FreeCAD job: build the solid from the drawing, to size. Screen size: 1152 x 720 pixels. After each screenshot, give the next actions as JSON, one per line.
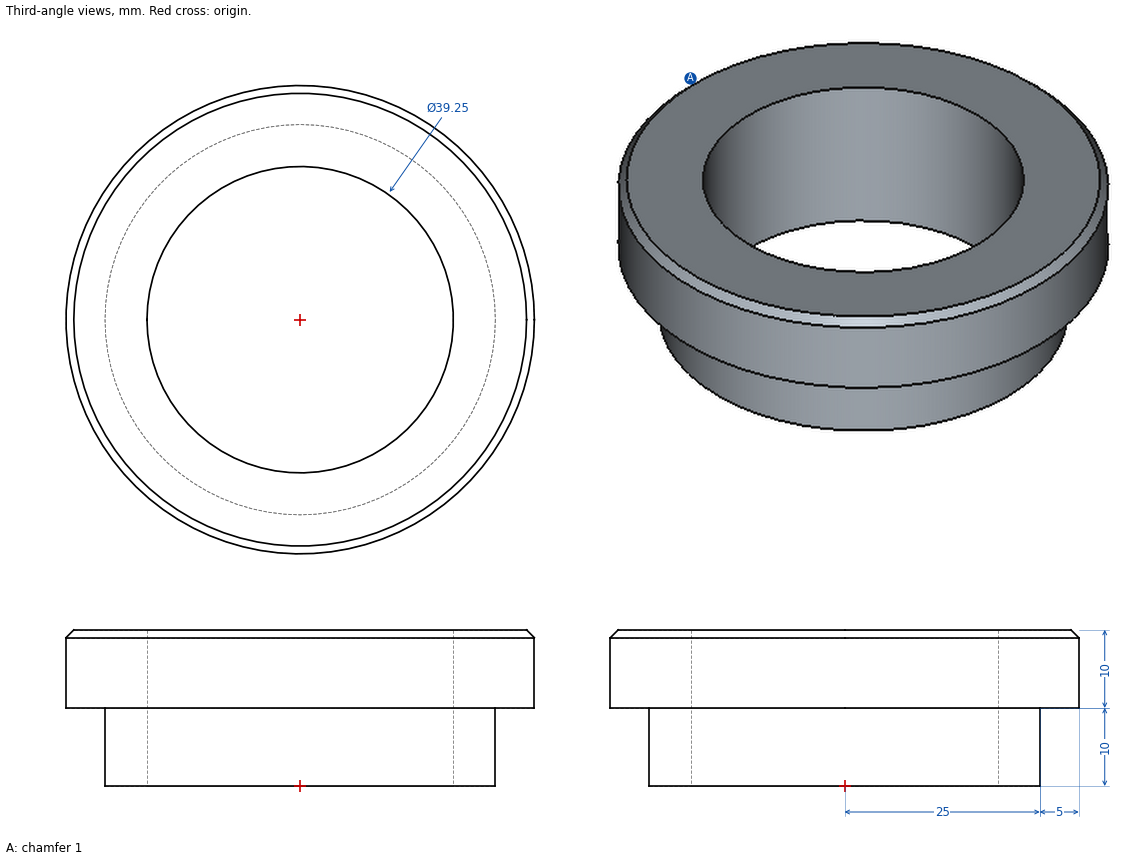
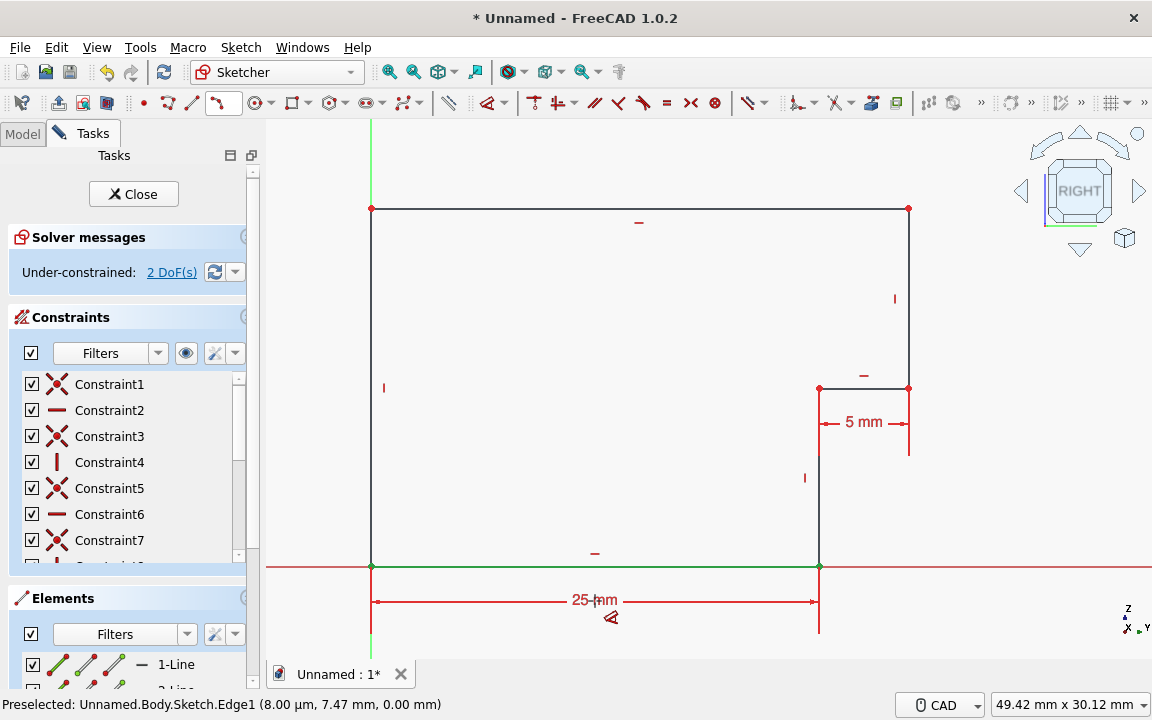
{"action": "left_click", "coordinate": [819, 513]}
{"action": "left_click", "coordinate": [853, 478]}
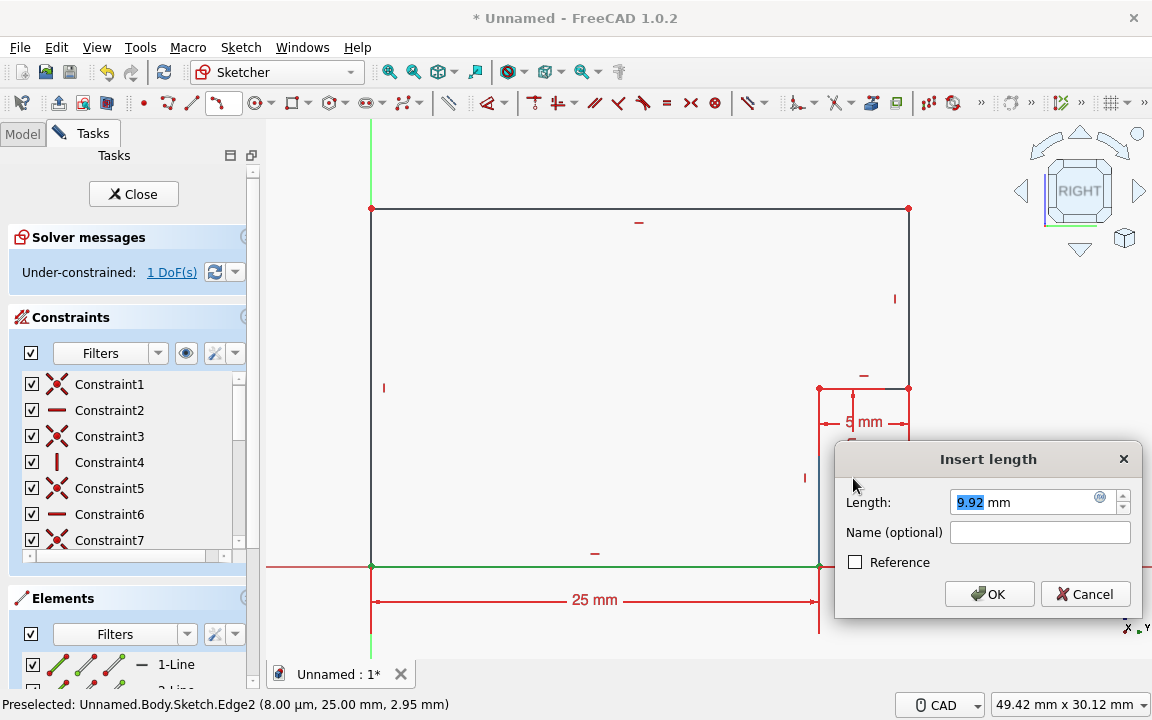
{"action": "type", "text": "10"}
{"action": "key", "text": "Return"}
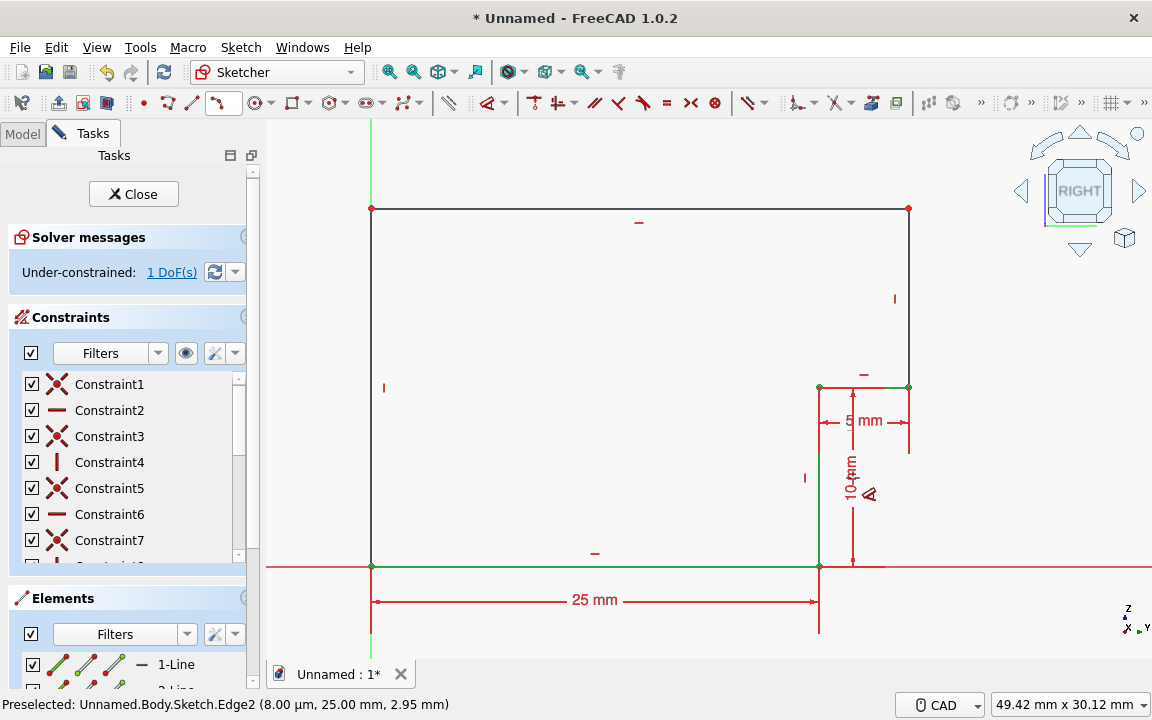
{"action": "left_click", "coordinate": [909, 334]}
{"action": "left_click", "coordinate": [943, 298]}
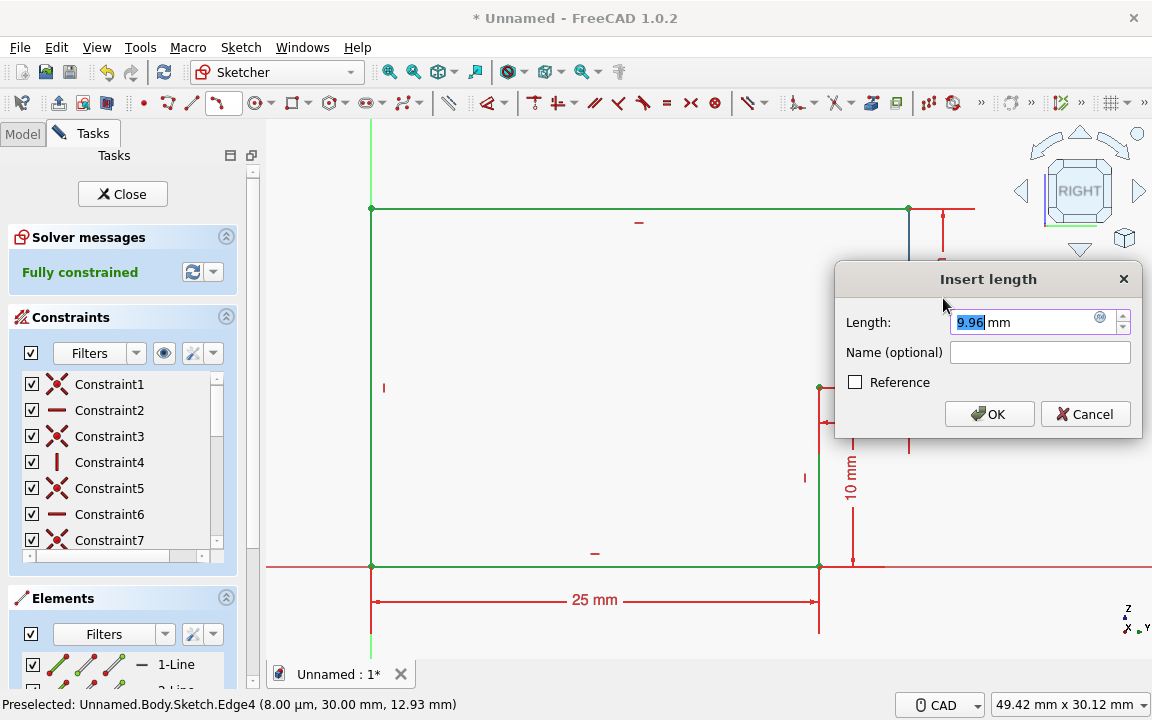
{"action": "type", "text": "10"}
{"action": "key", "text": "Return"}
{"action": "key", "text": "Escape"}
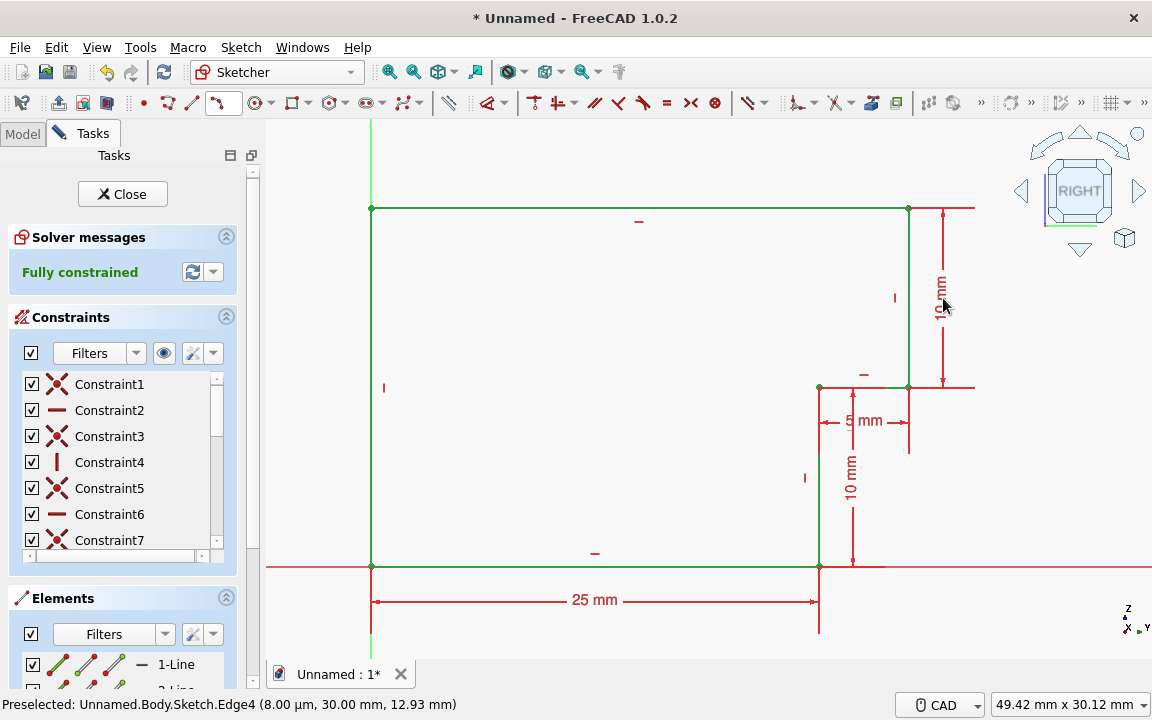
{"action": "left_click", "coordinate": [123, 194]}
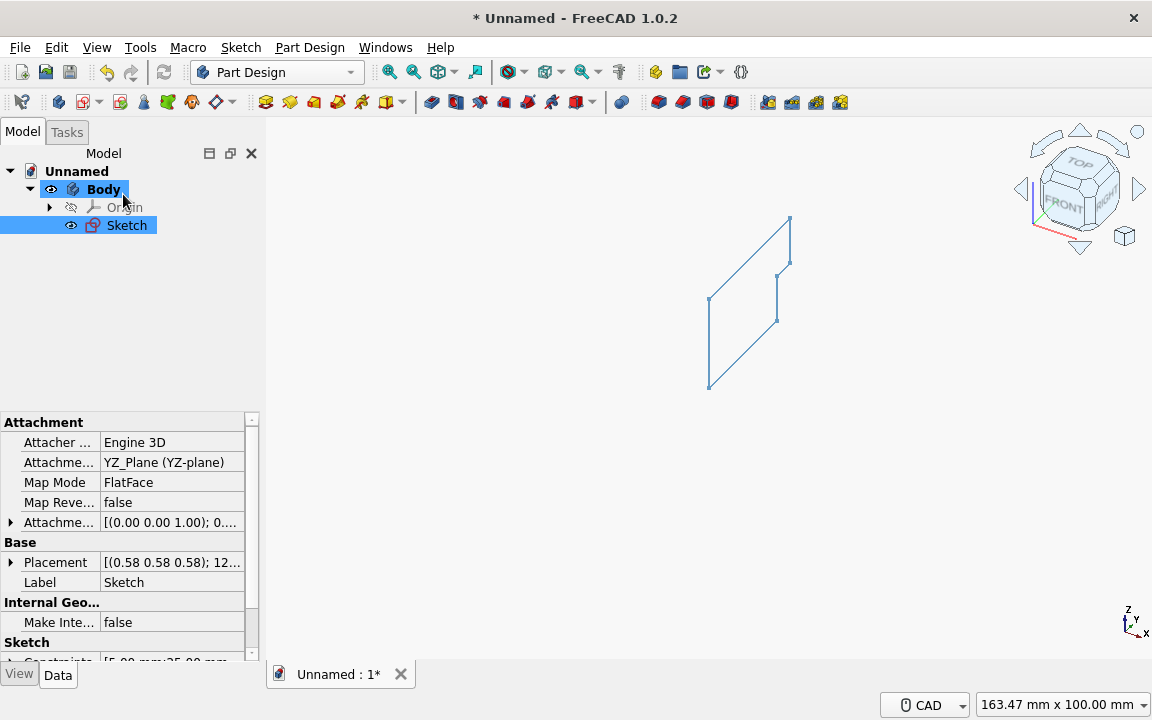
{"action": "left_click", "coordinate": [290, 102]}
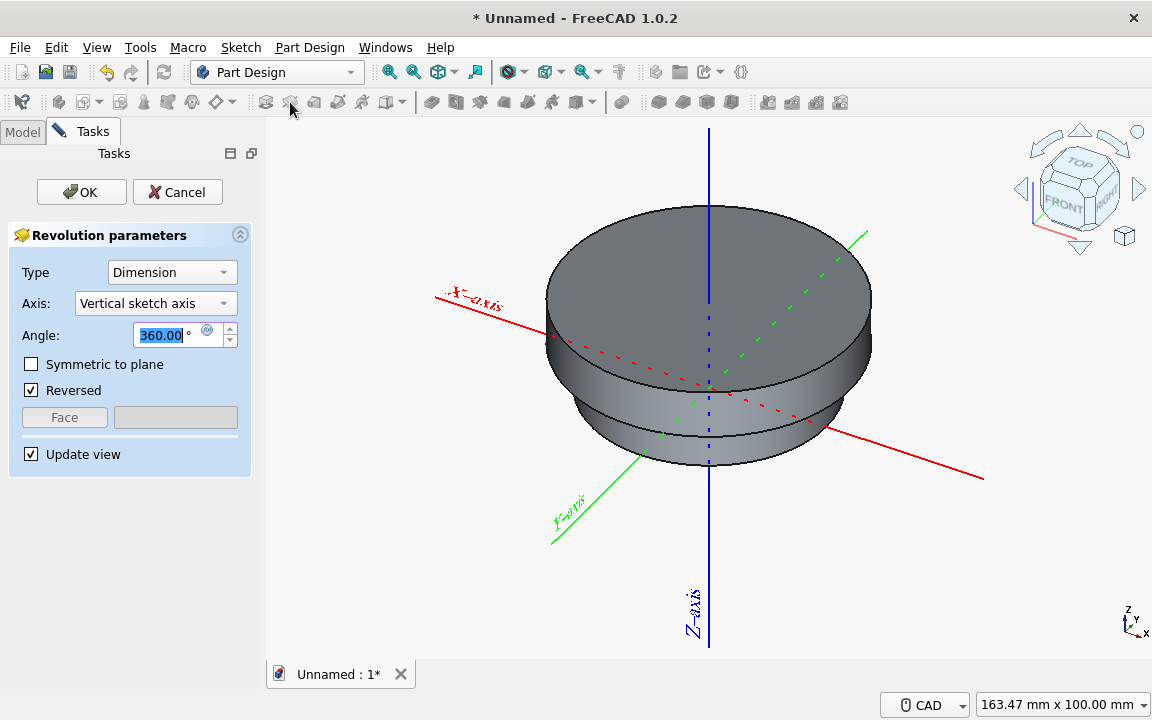
{"action": "left_click", "coordinate": [82, 192]}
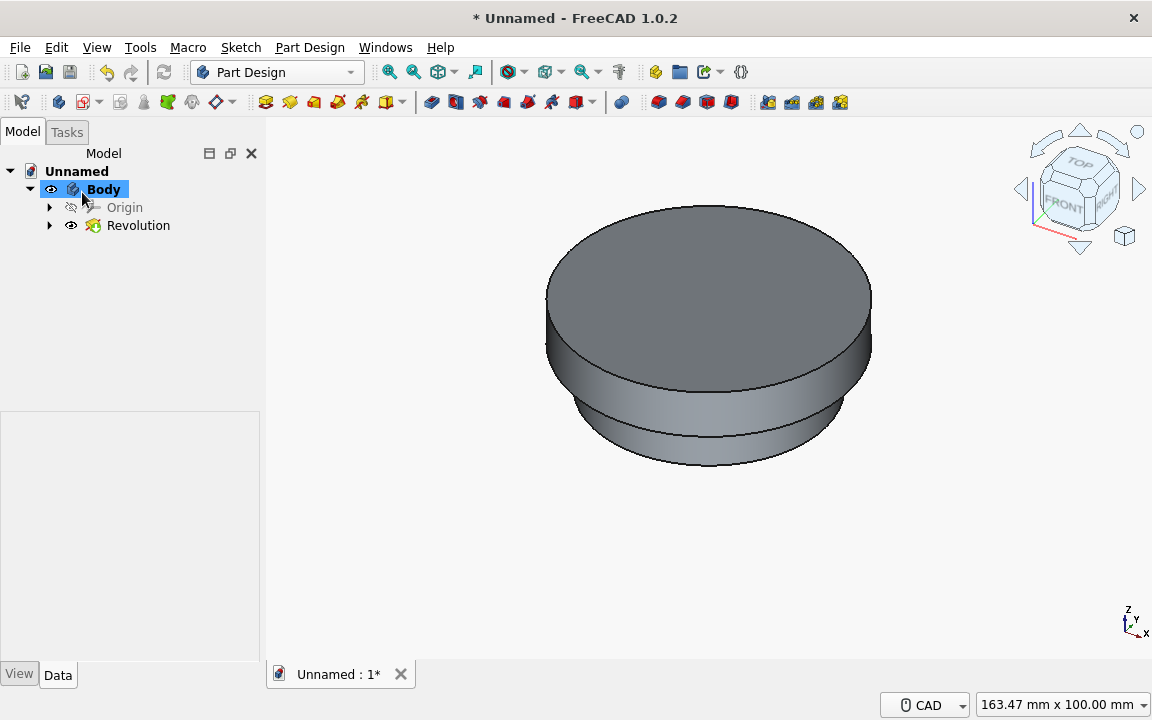
{"action": "left_click", "coordinate": [709, 298]}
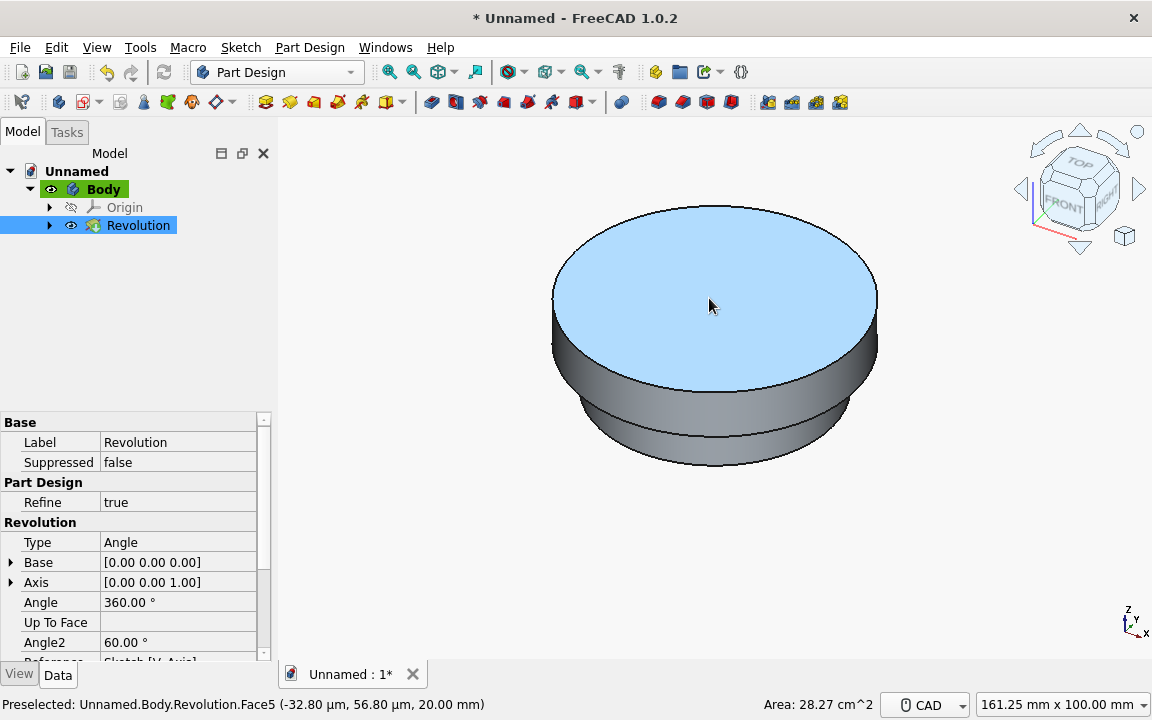
{"action": "left_click", "coordinate": [84, 102]}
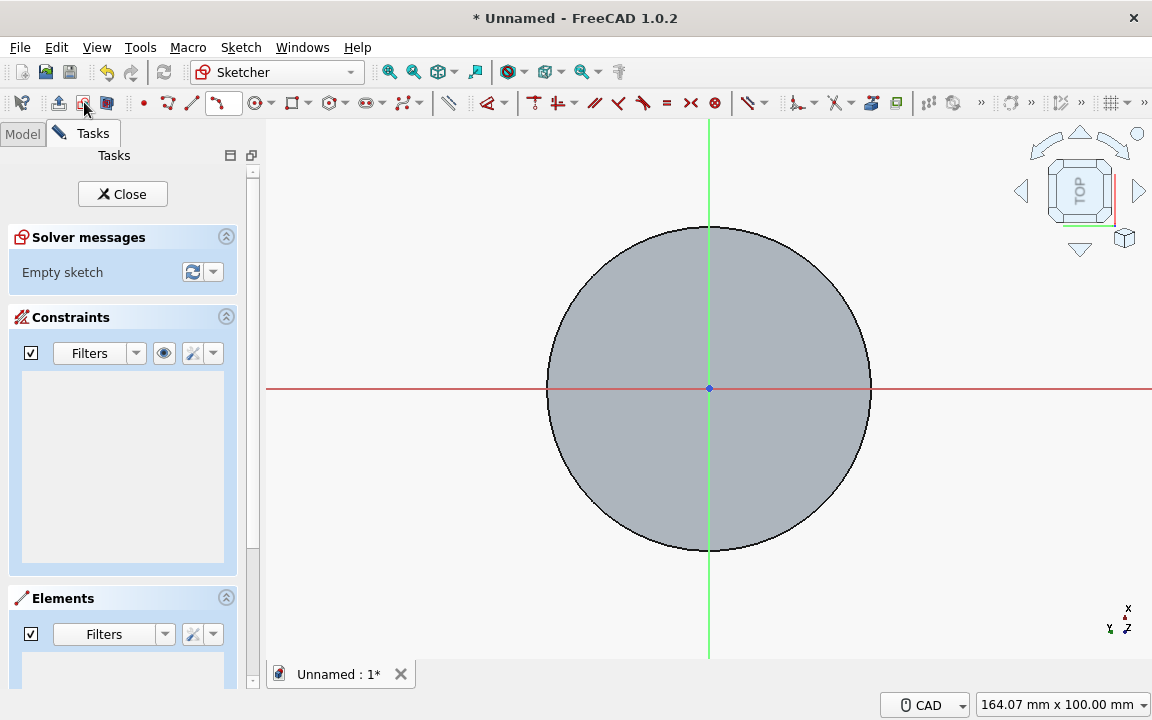
{"action": "scroll", "coordinate": [848, 389], "scroll_direction": "up", "scroll_amount": 2}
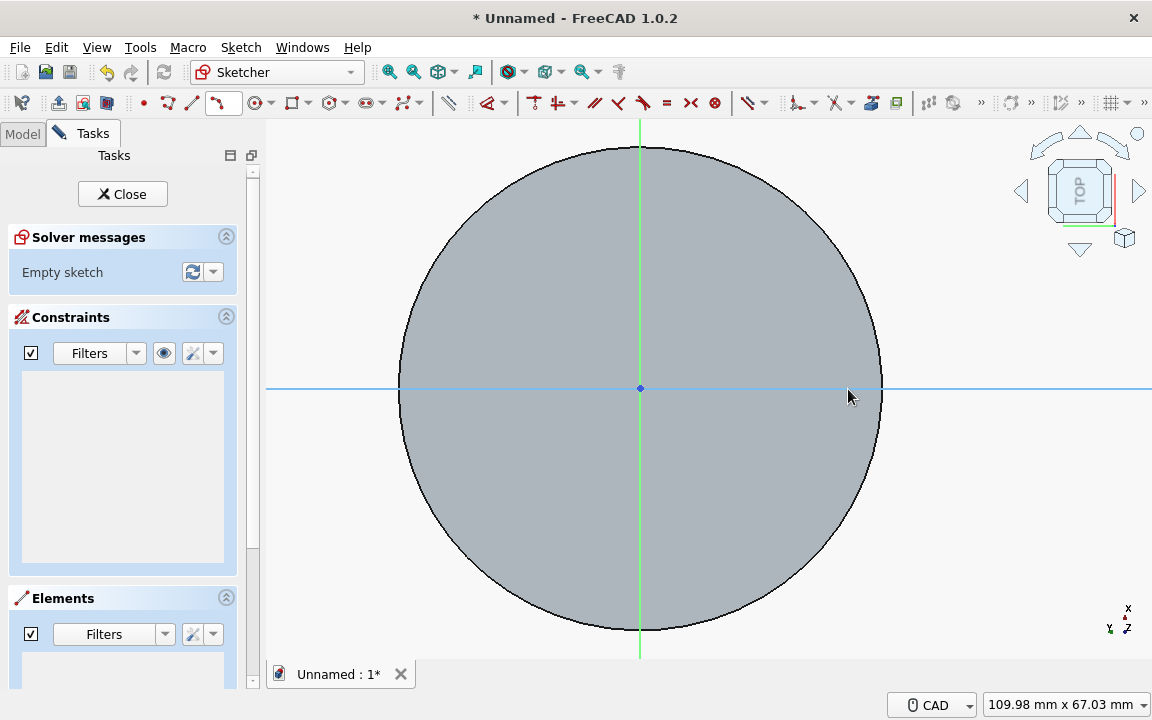
{"action": "left_click", "coordinate": [256, 104]}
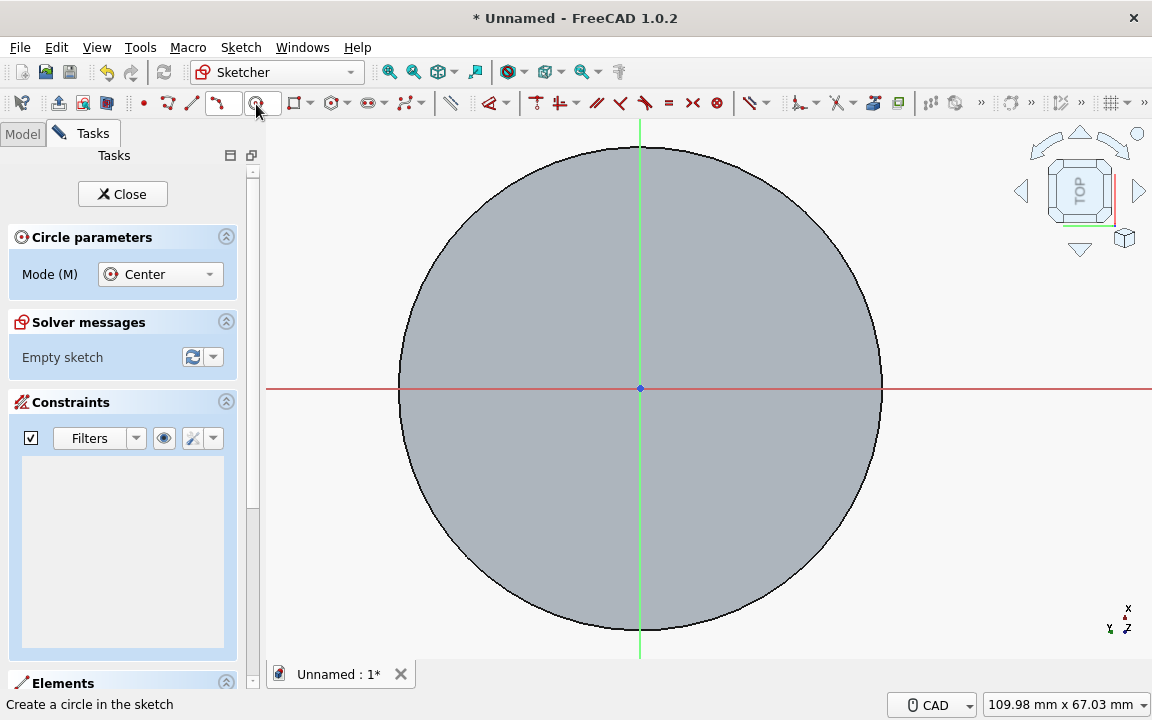
{"action": "left_click", "coordinate": [640, 389]}
{"action": "left_click", "coordinate": [752, 277]}
{"action": "key", "text": "Escape"}